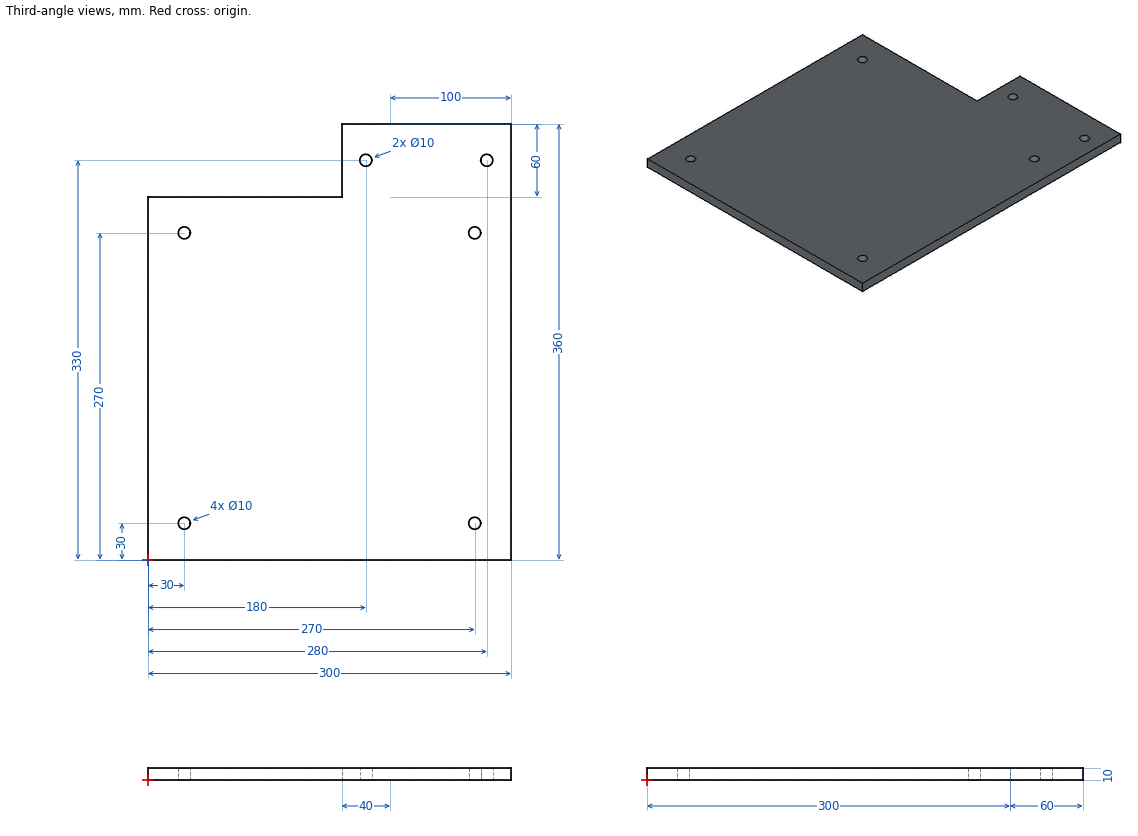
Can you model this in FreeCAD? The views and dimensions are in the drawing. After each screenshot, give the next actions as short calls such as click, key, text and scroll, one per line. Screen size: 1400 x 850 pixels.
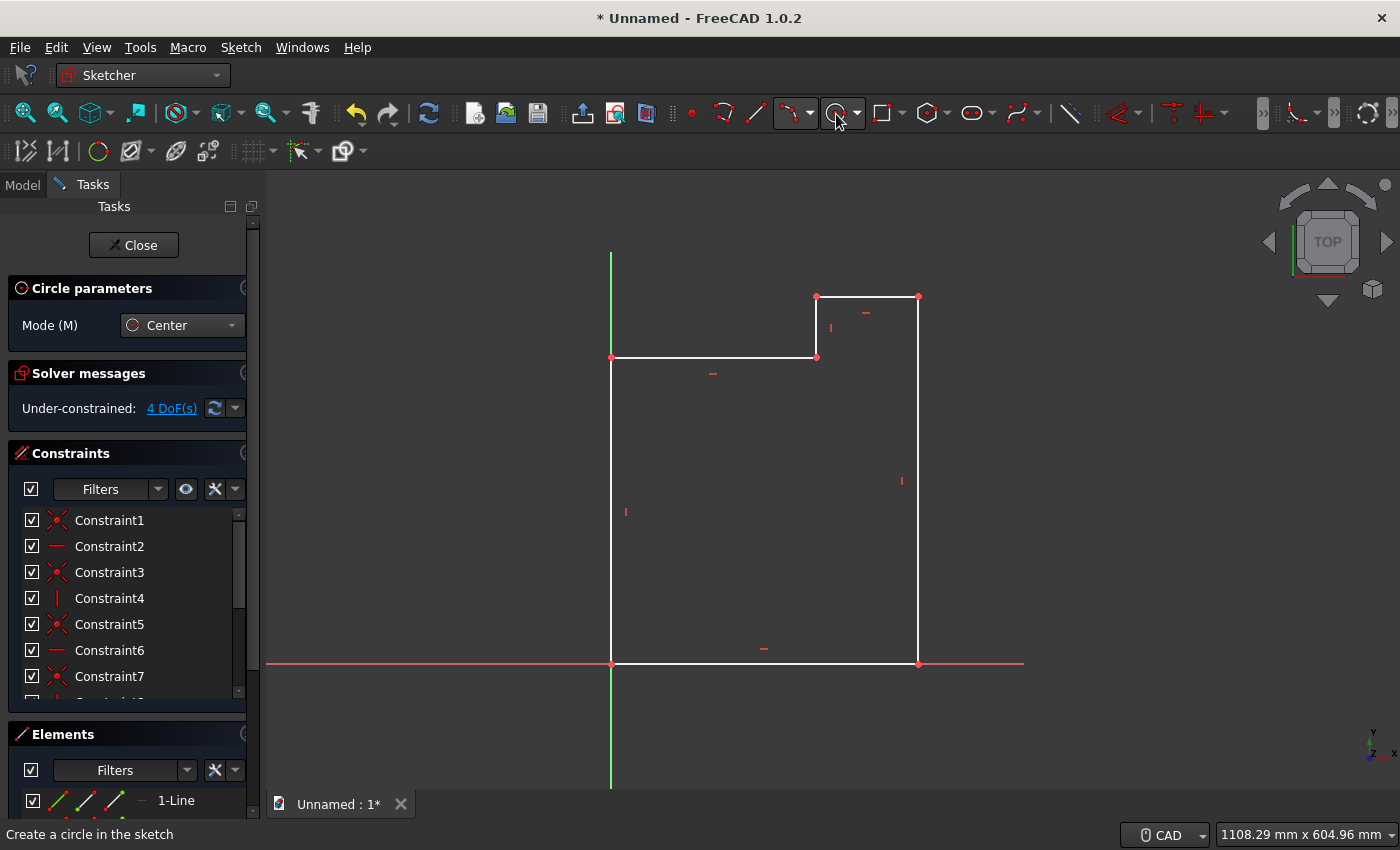
scroll(642, 634, up, 8)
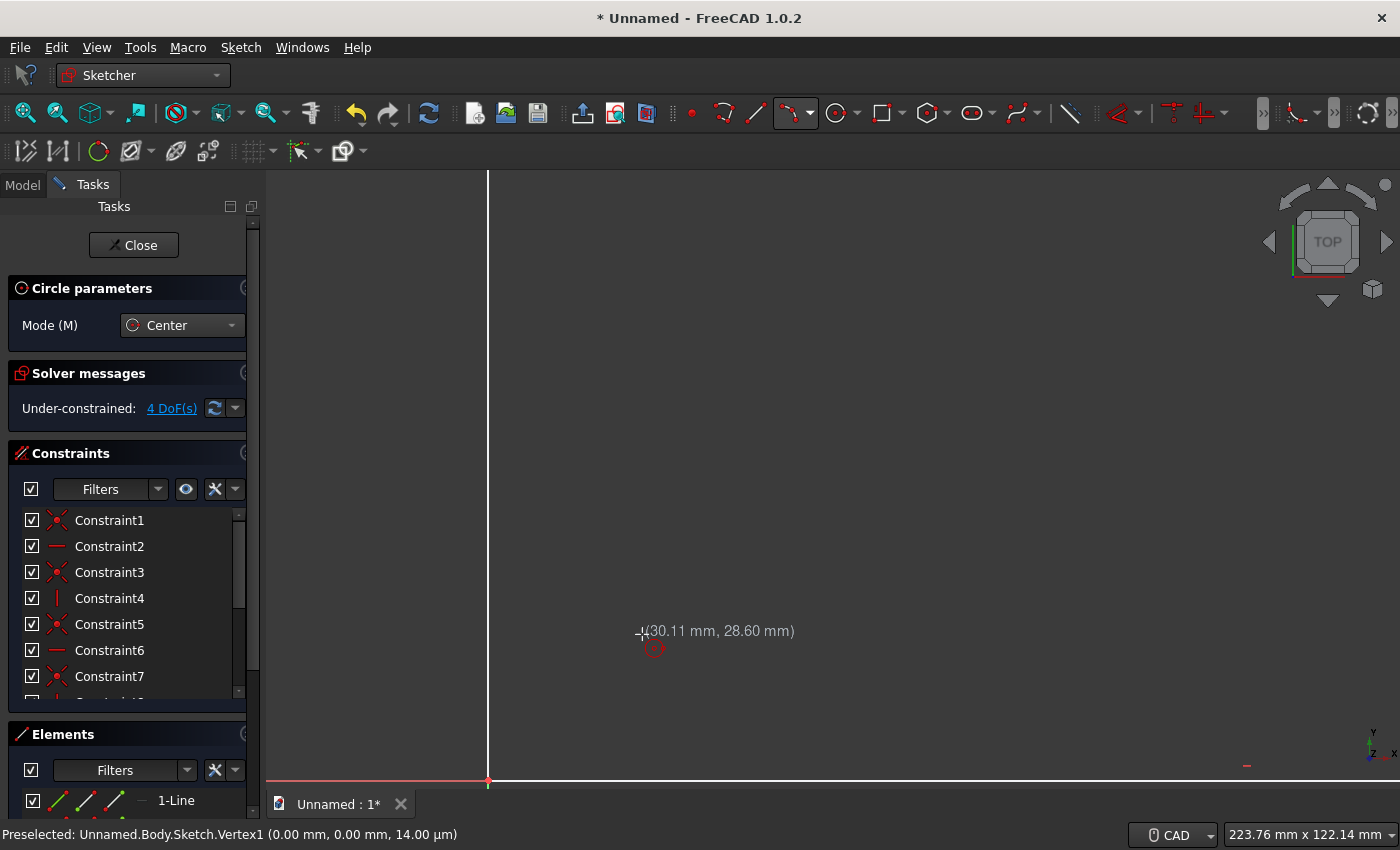
scroll(642, 634, down, 8)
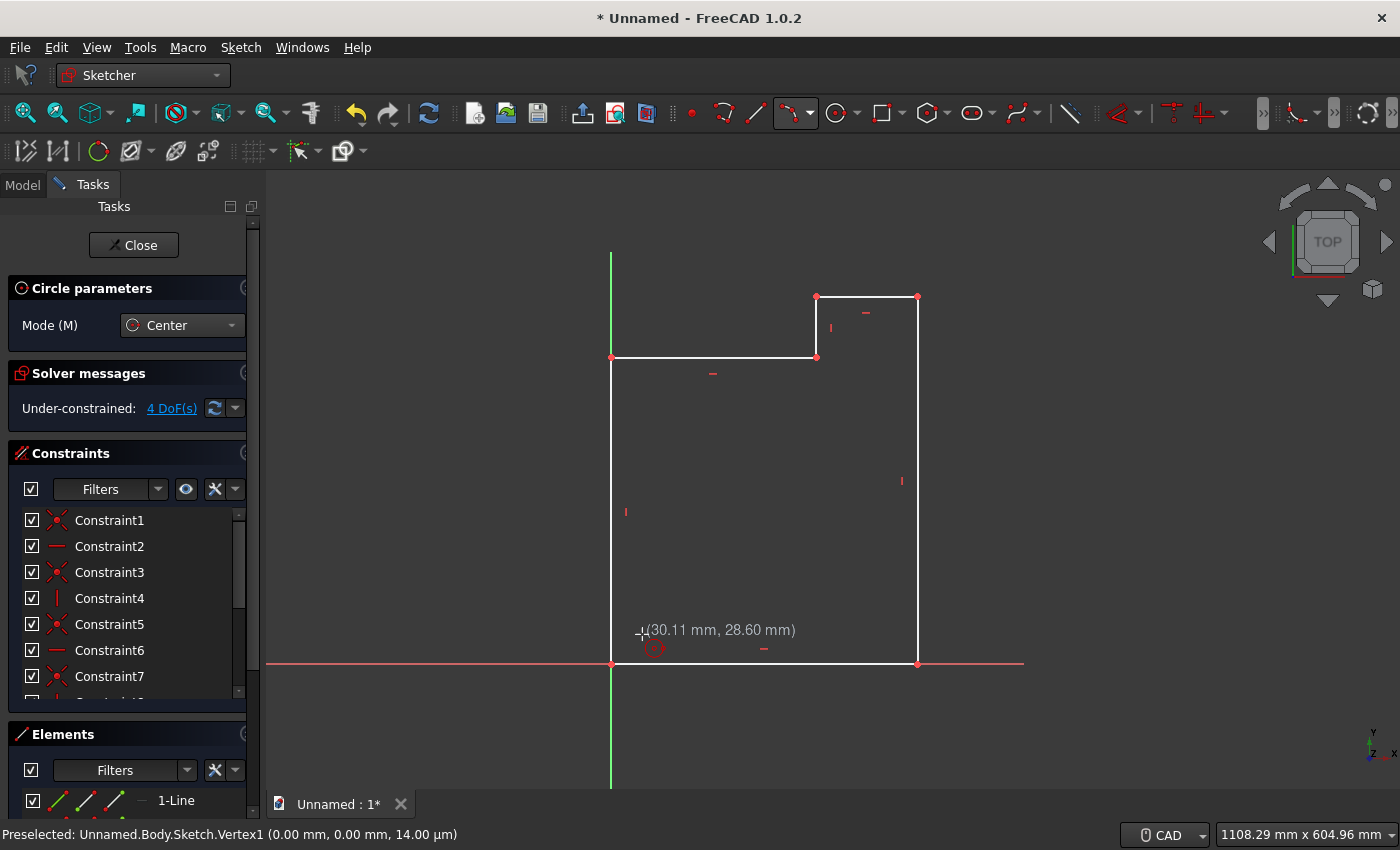
click(642, 634)
move(646, 630)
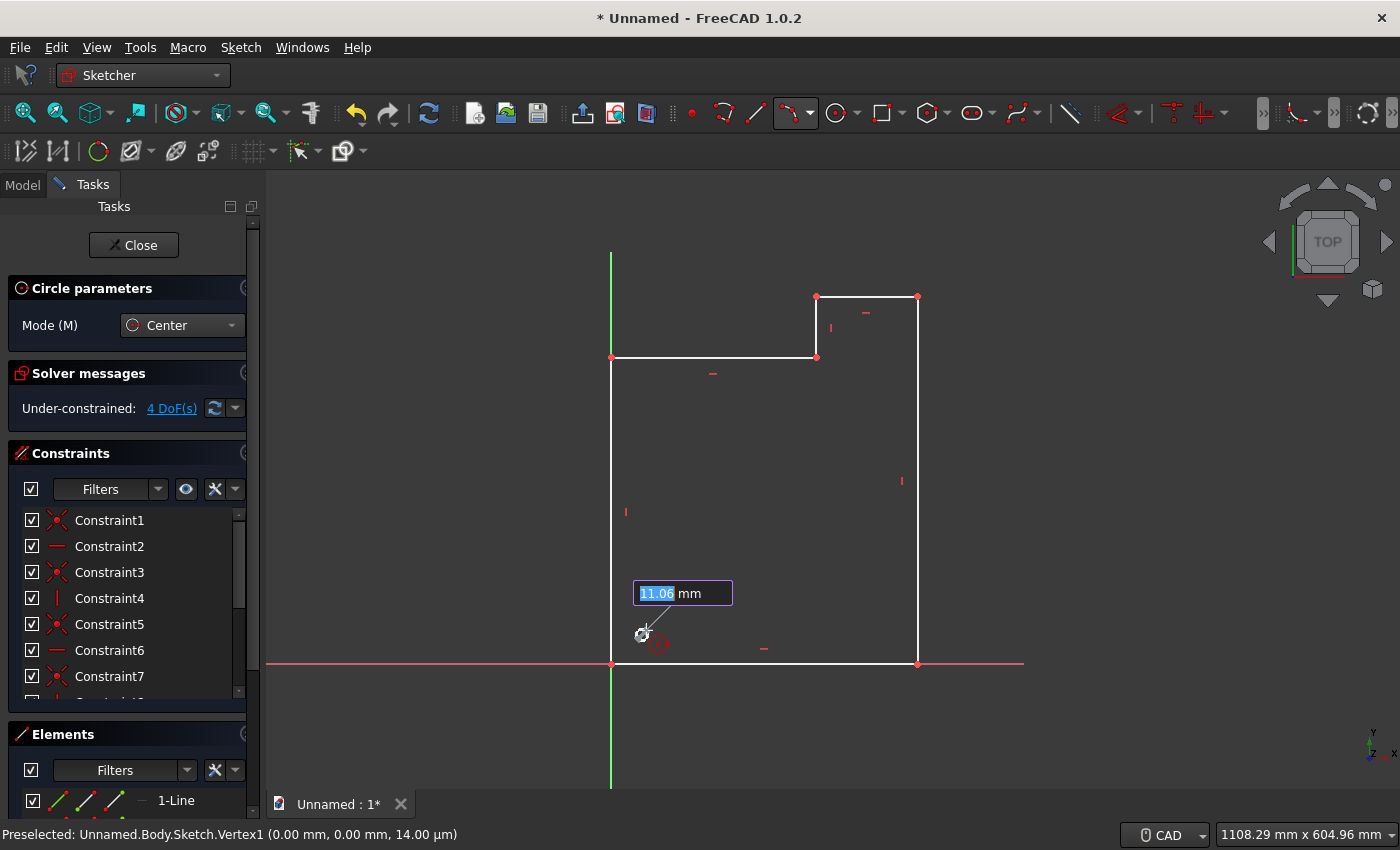
text(10)
key(Return)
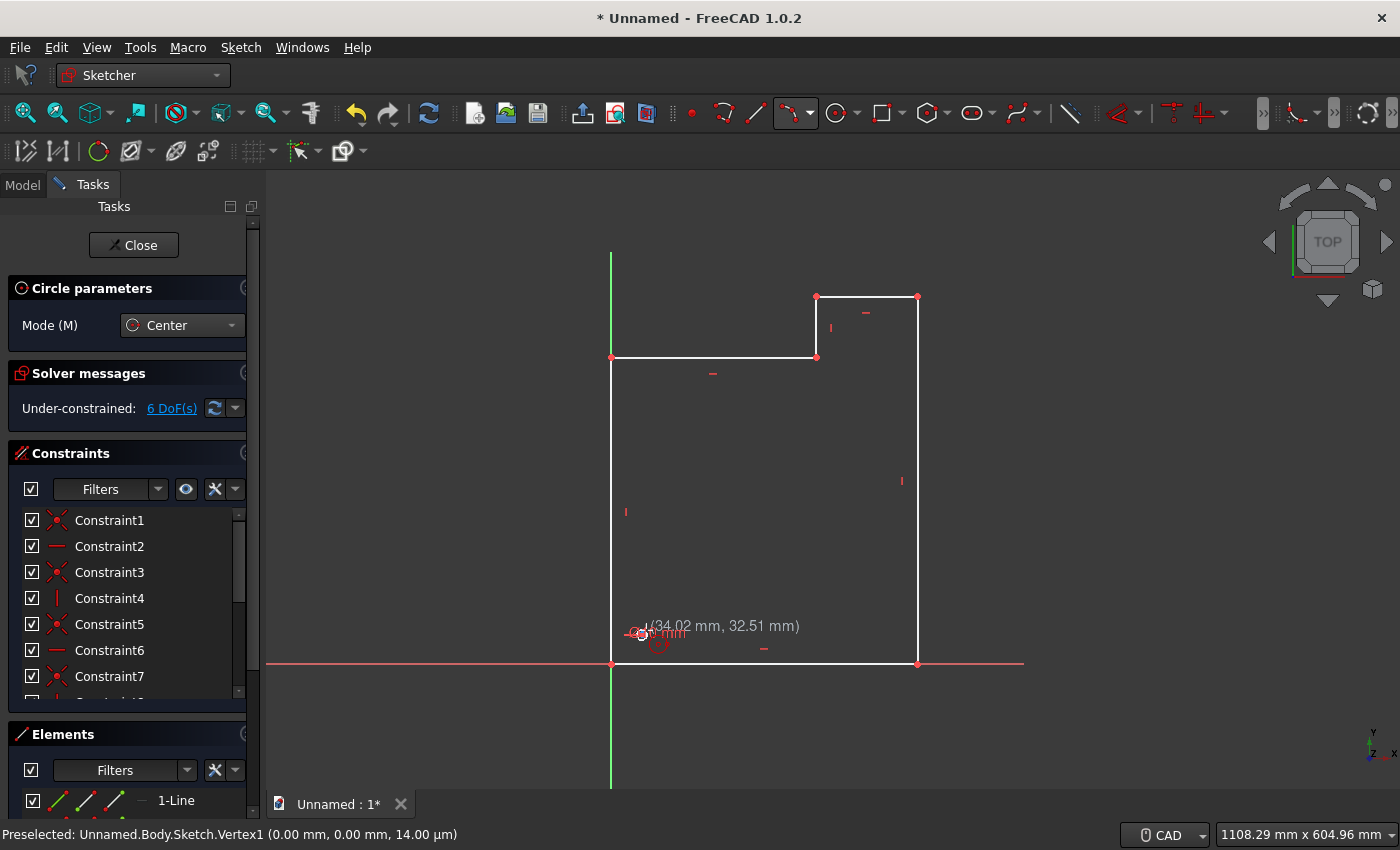
scroll(887, 634, up, 8)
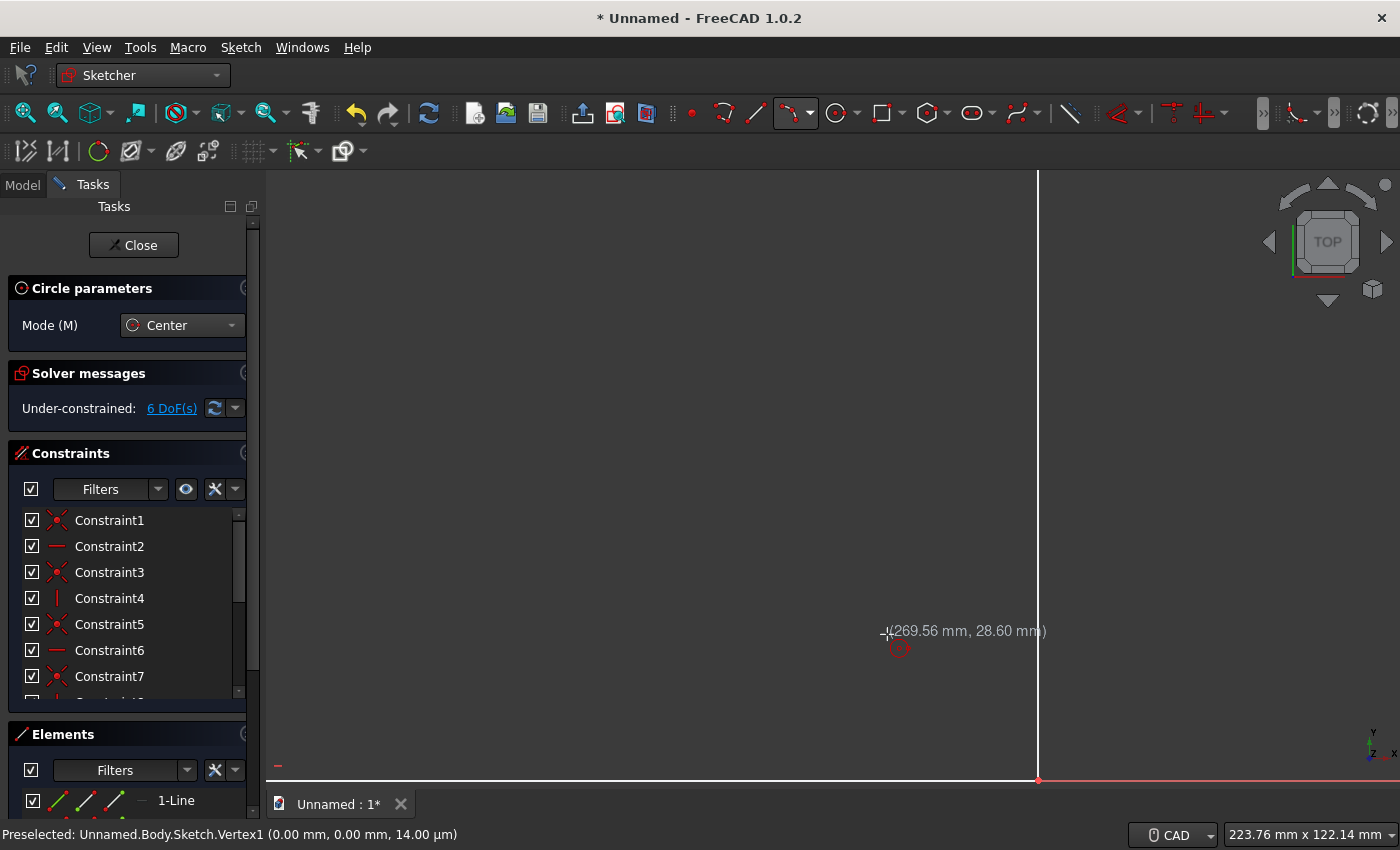
scroll(887, 634, down, 8)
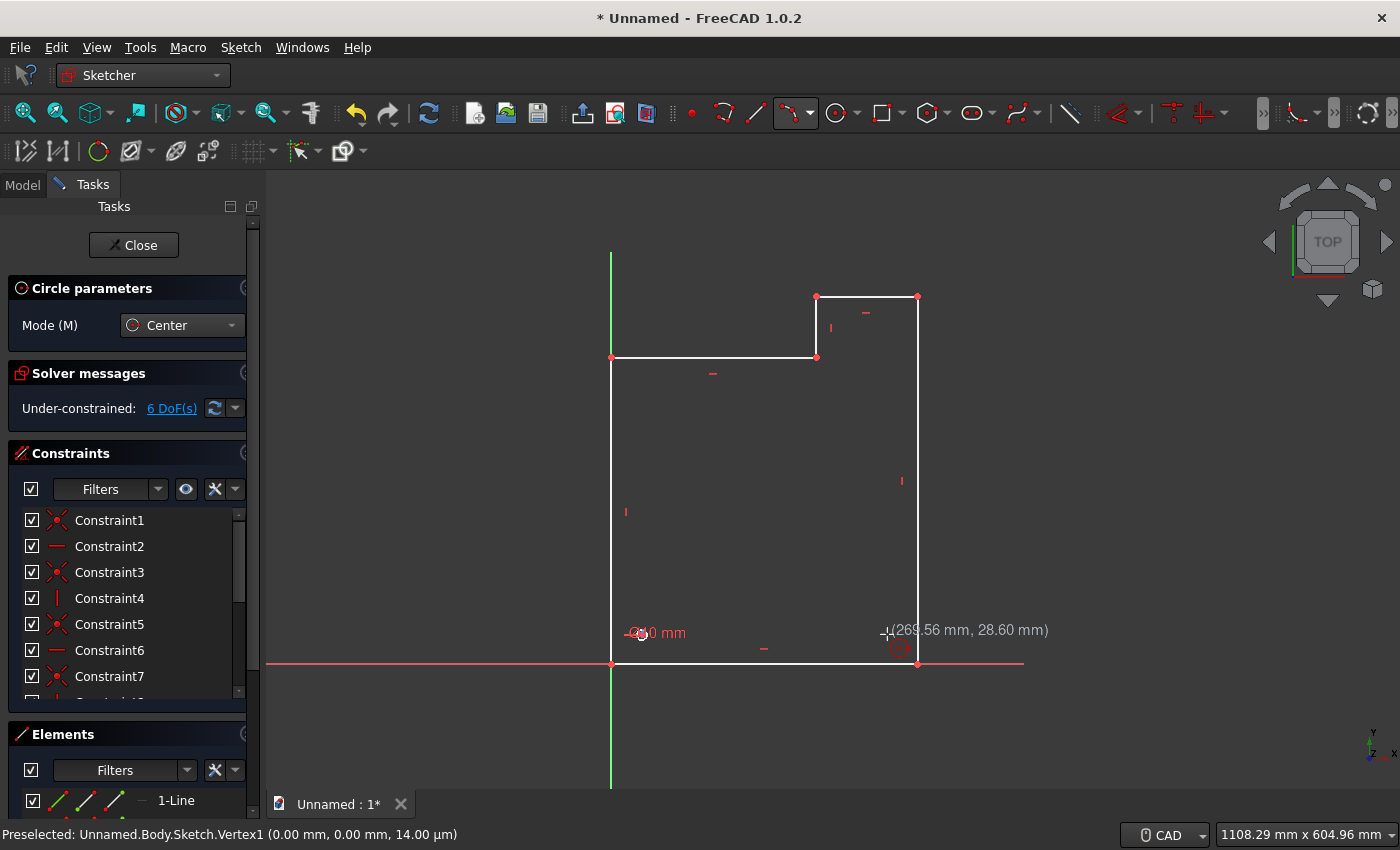
click(887, 634)
move(891, 630)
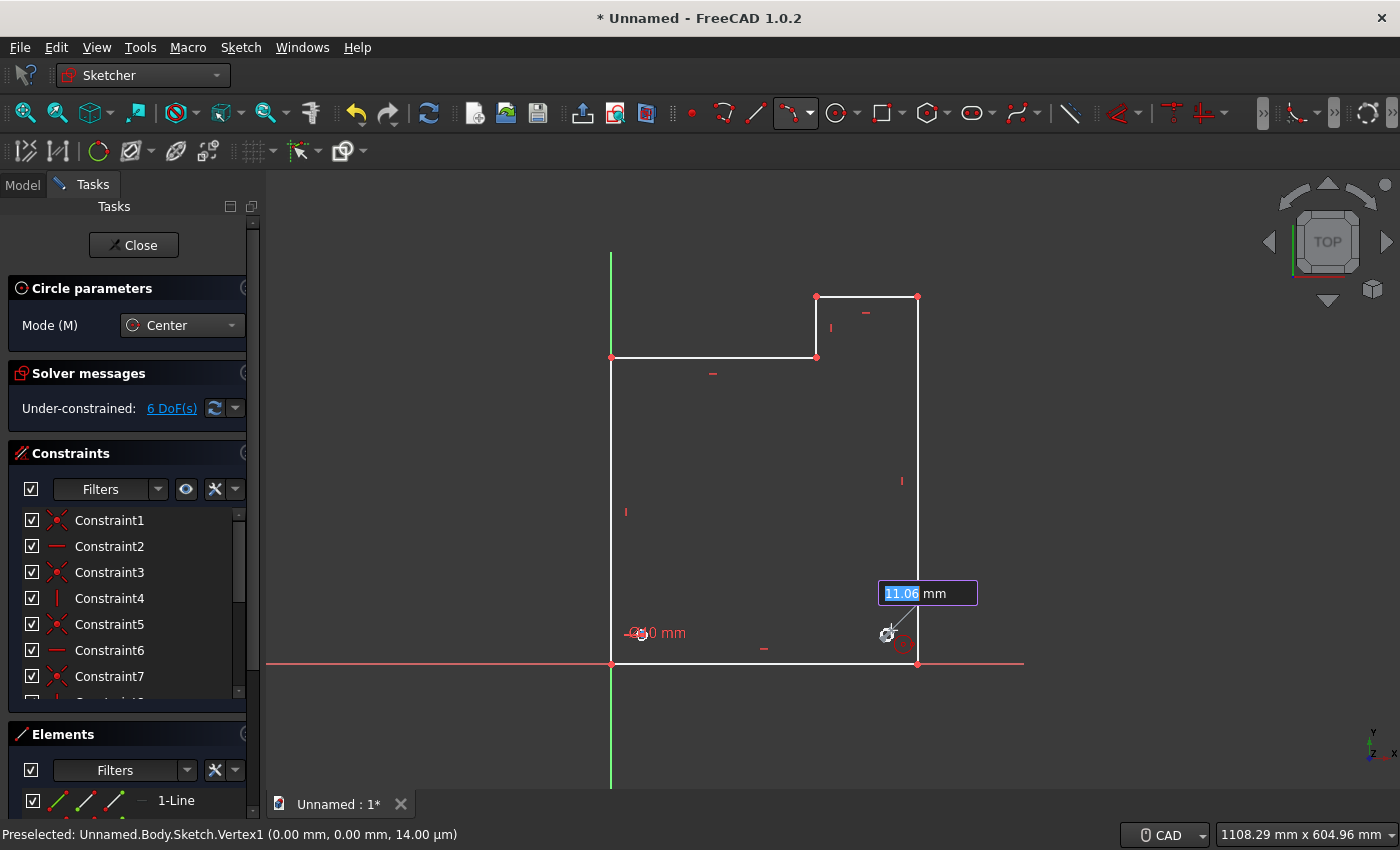
text(10)
key(Return)